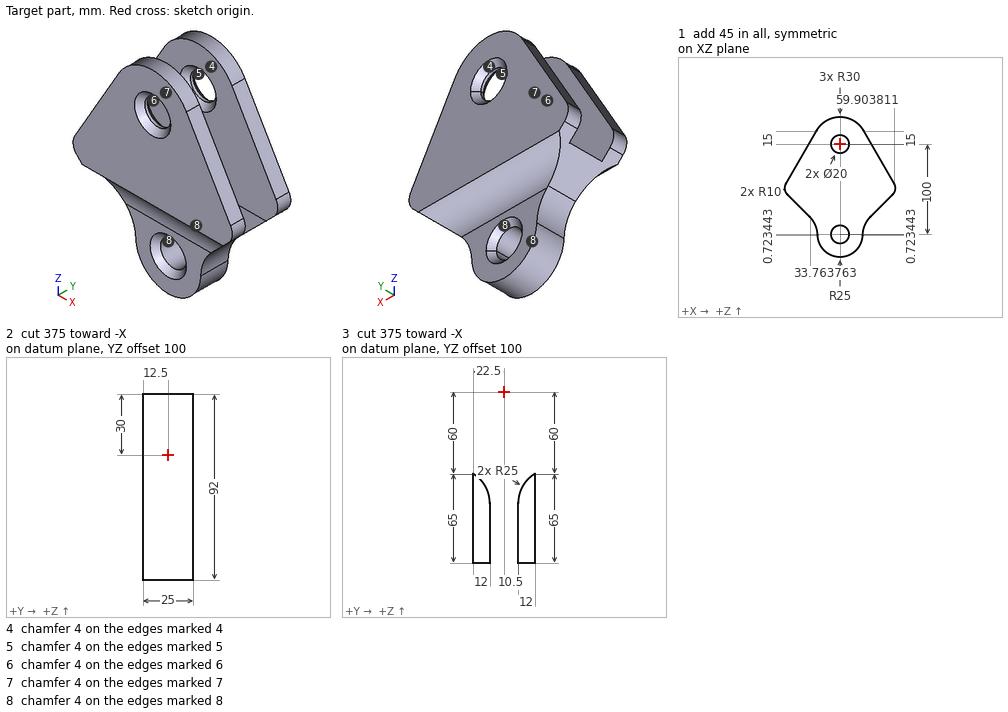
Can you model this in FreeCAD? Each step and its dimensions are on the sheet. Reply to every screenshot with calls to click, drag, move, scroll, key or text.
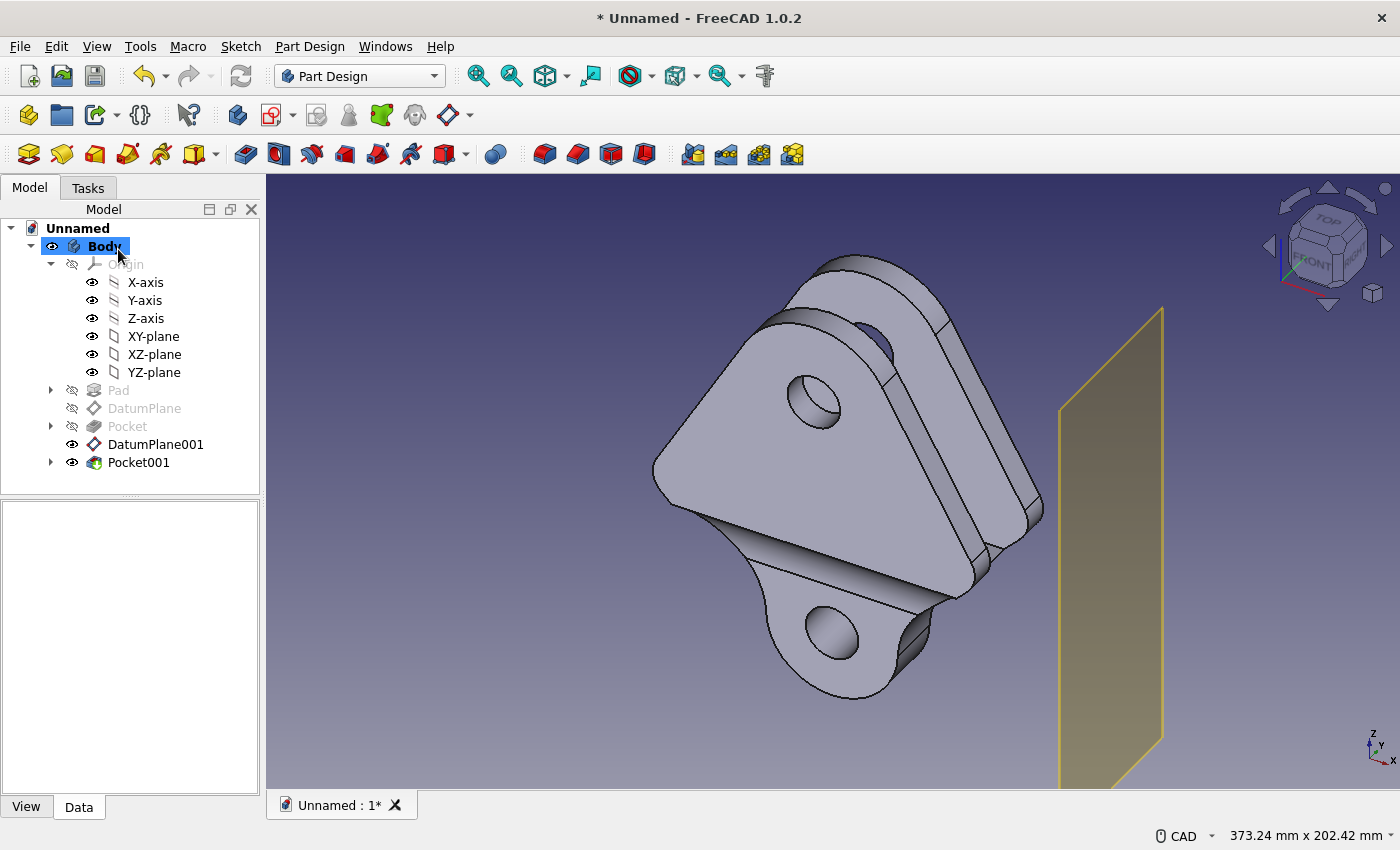
click(117, 444)
key(space)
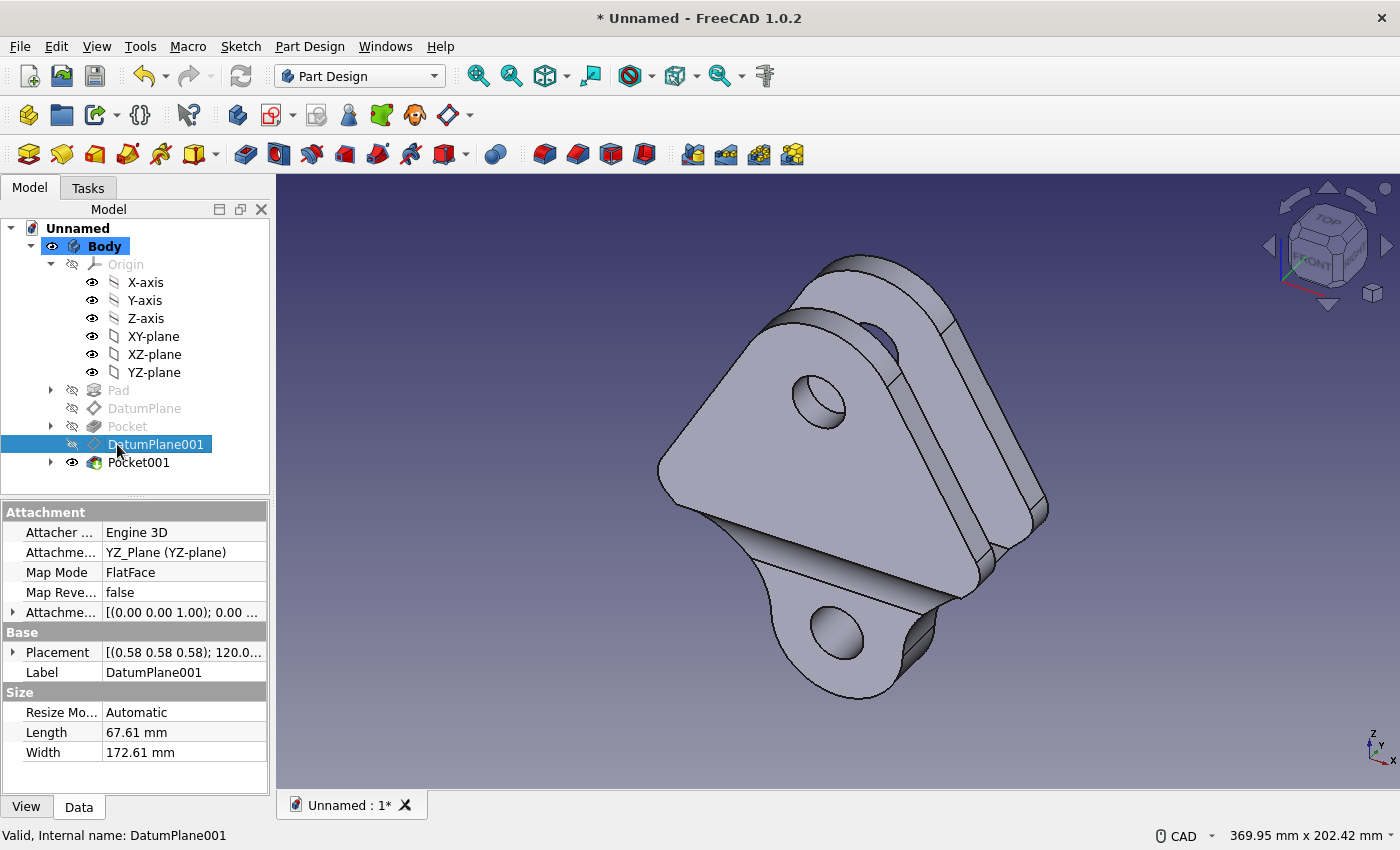
key(0)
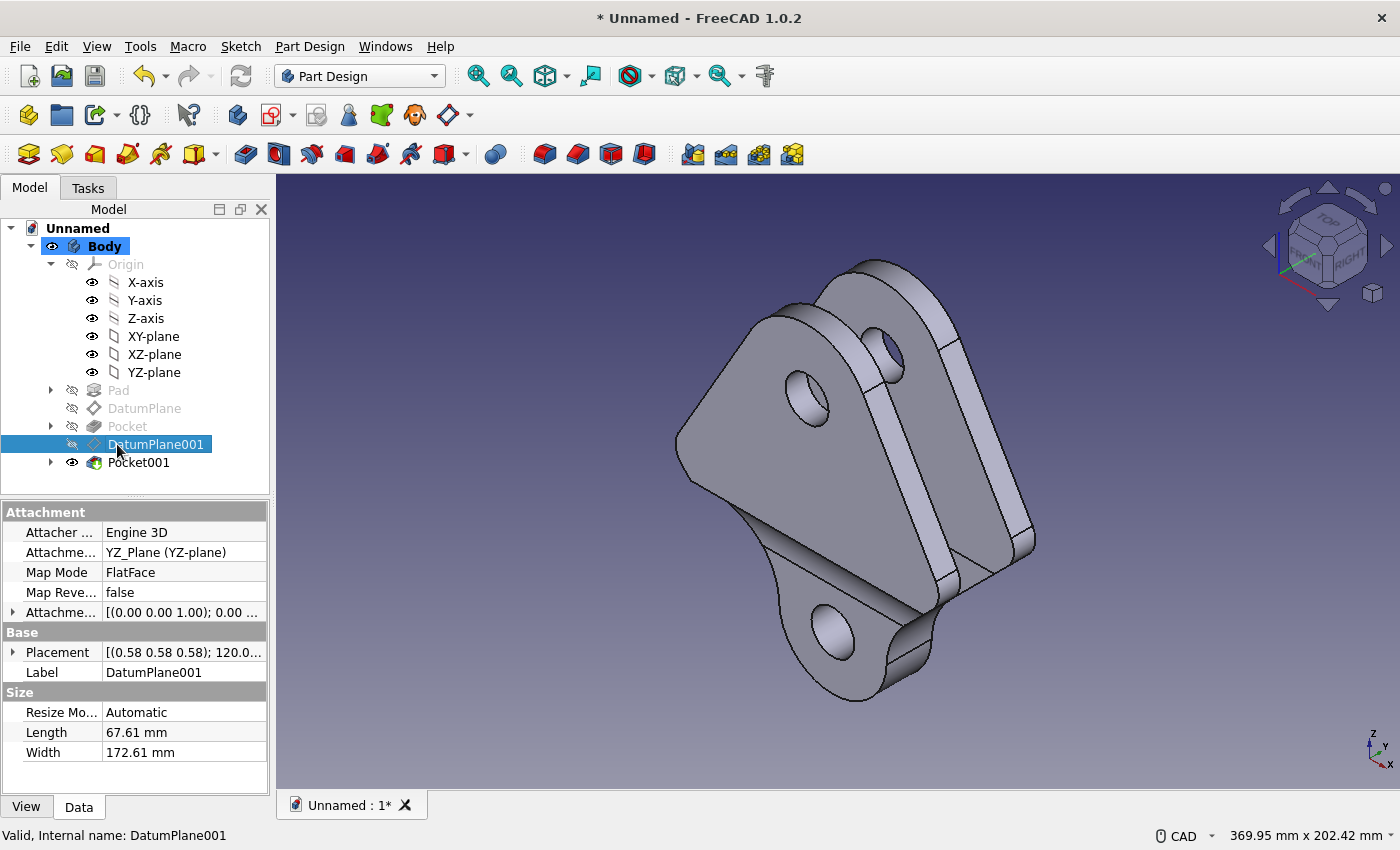
key(2)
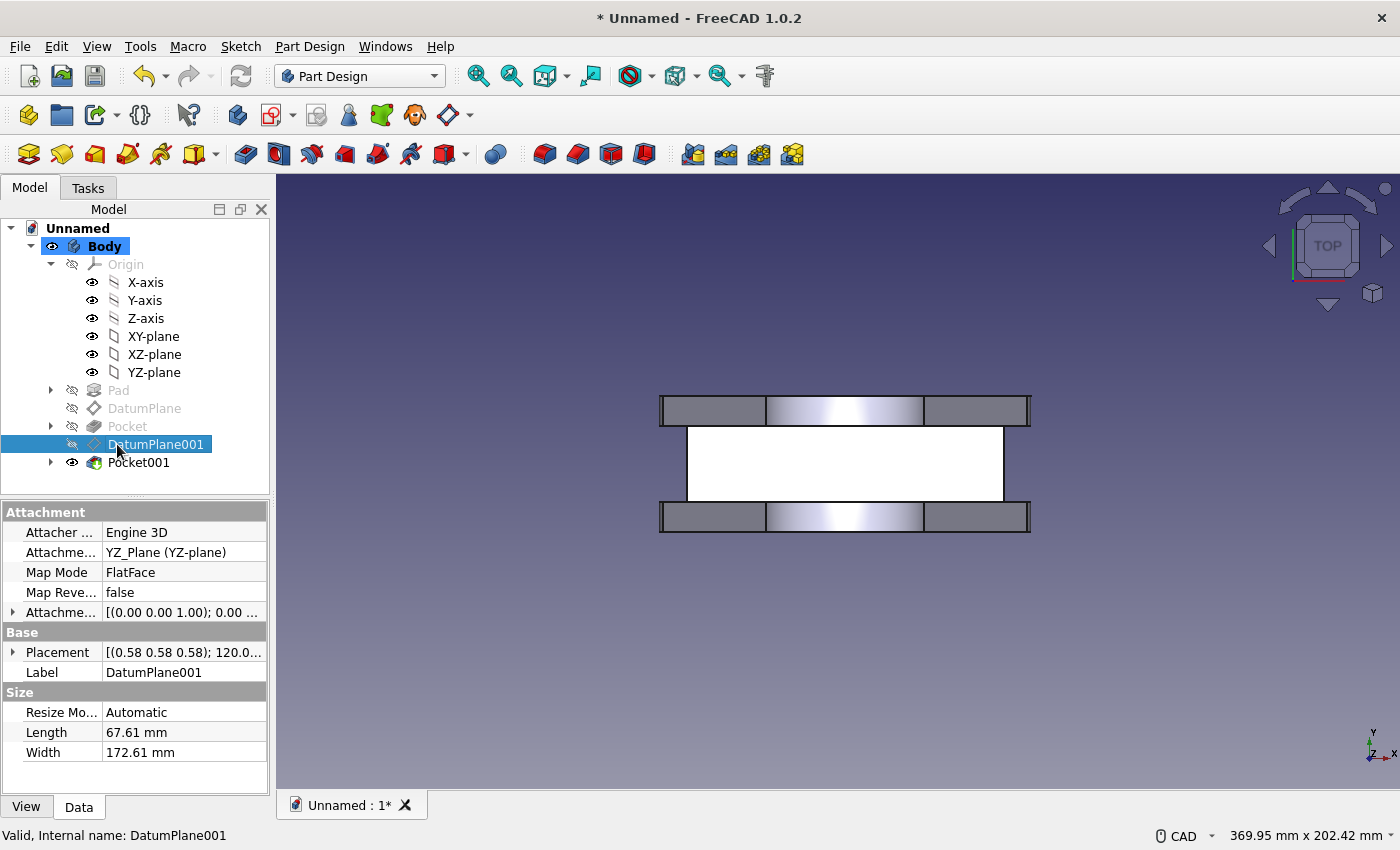
key(v)
key(f)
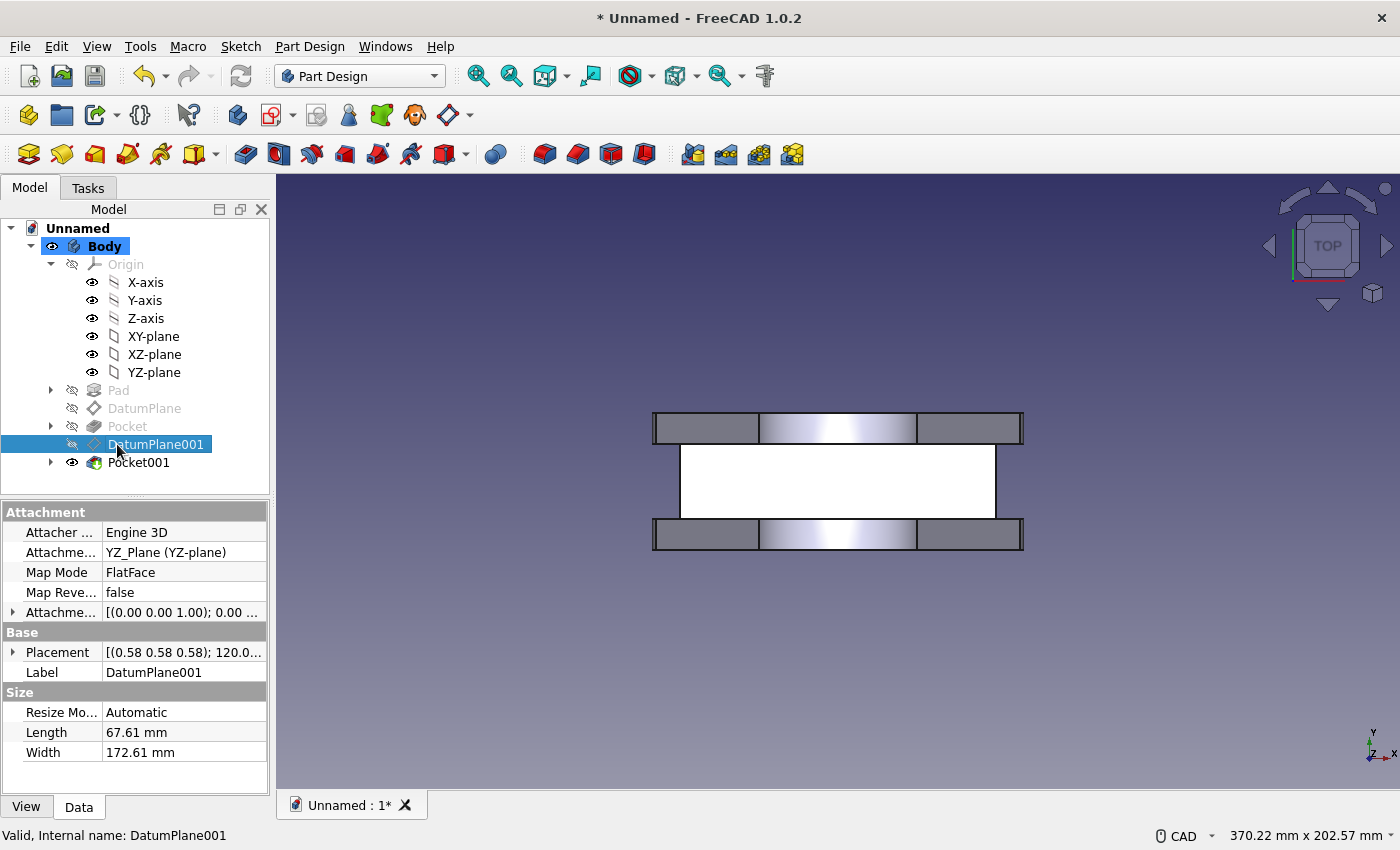
key(1)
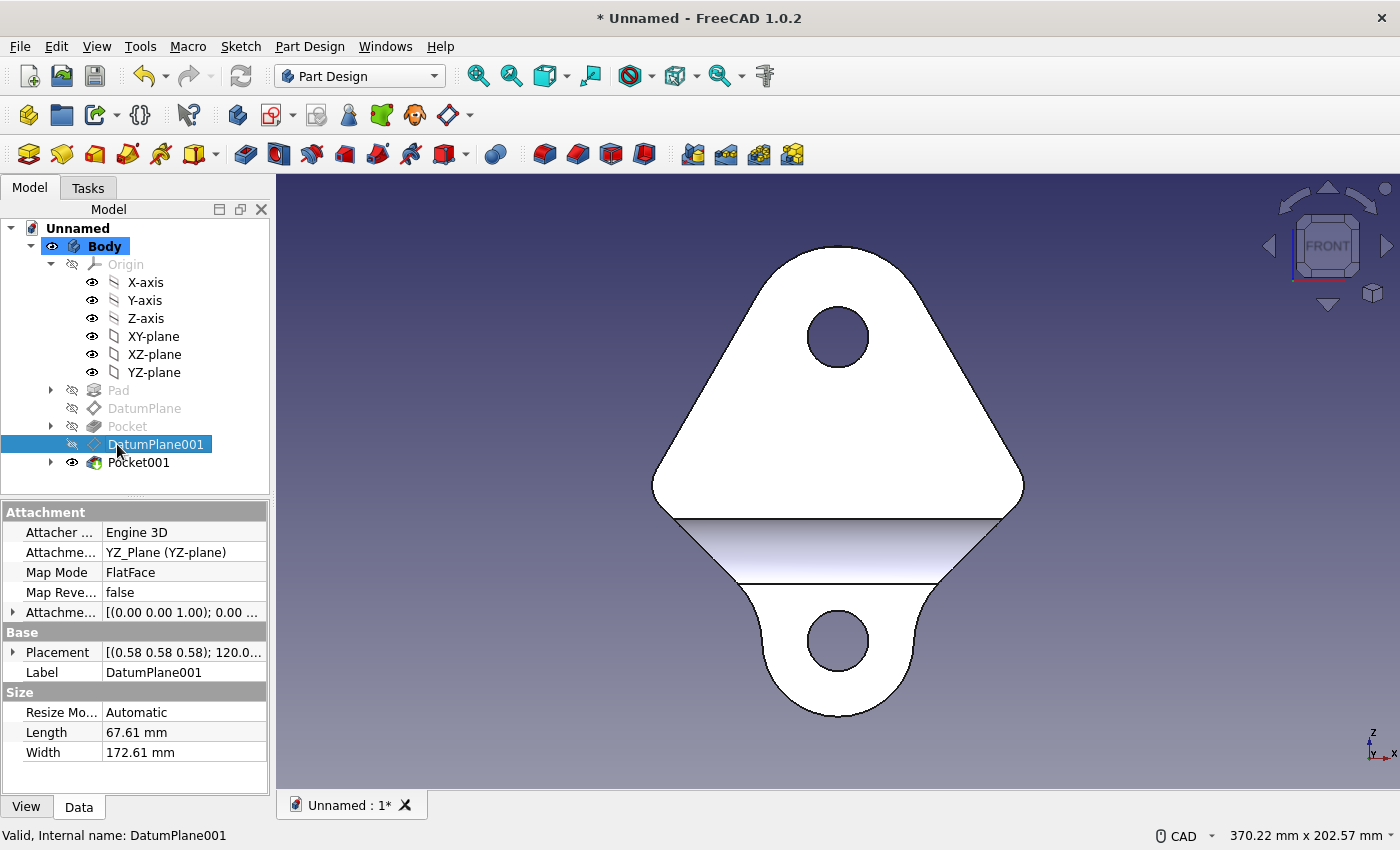
key(3)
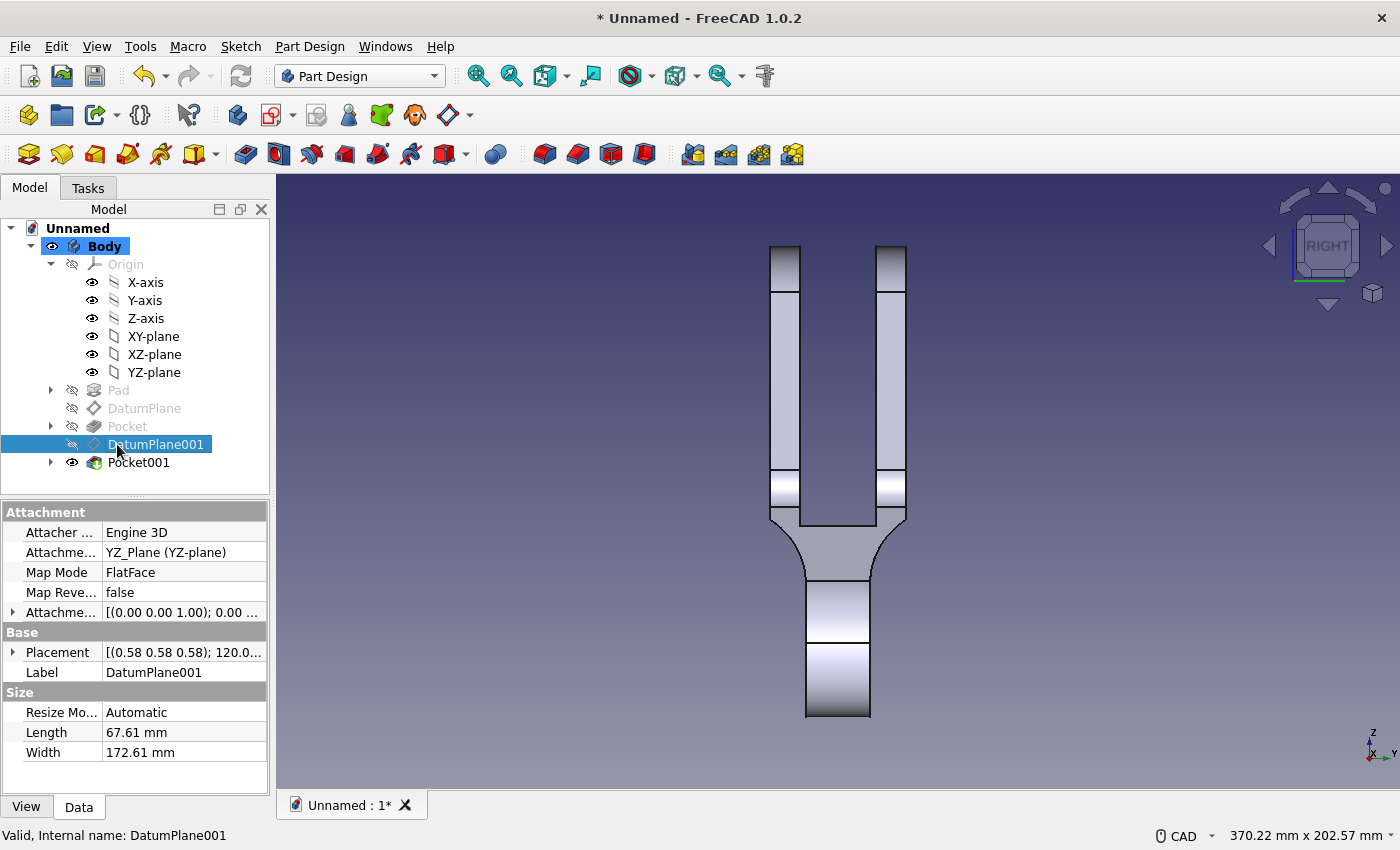
key(5)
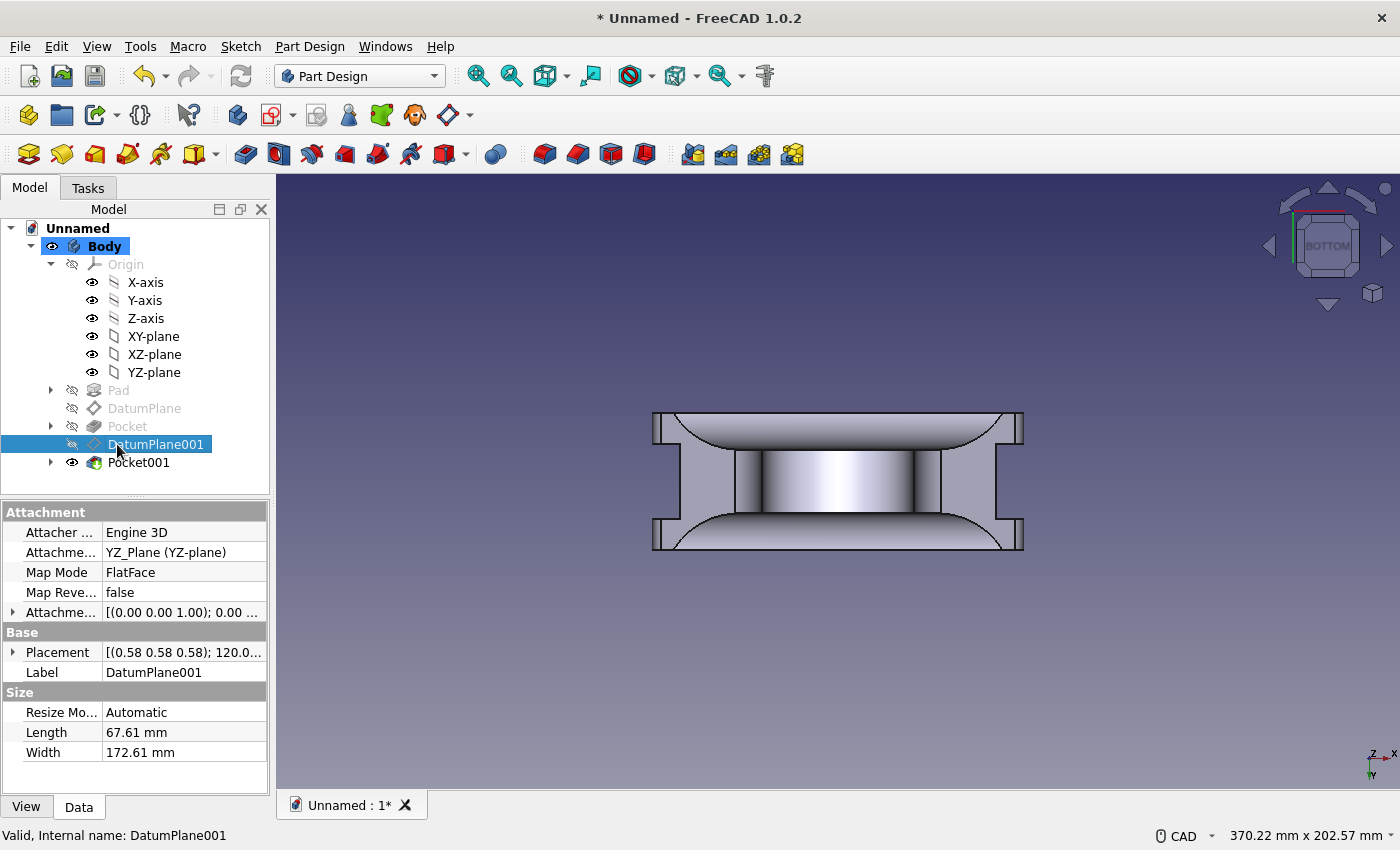
key(v)
key(f)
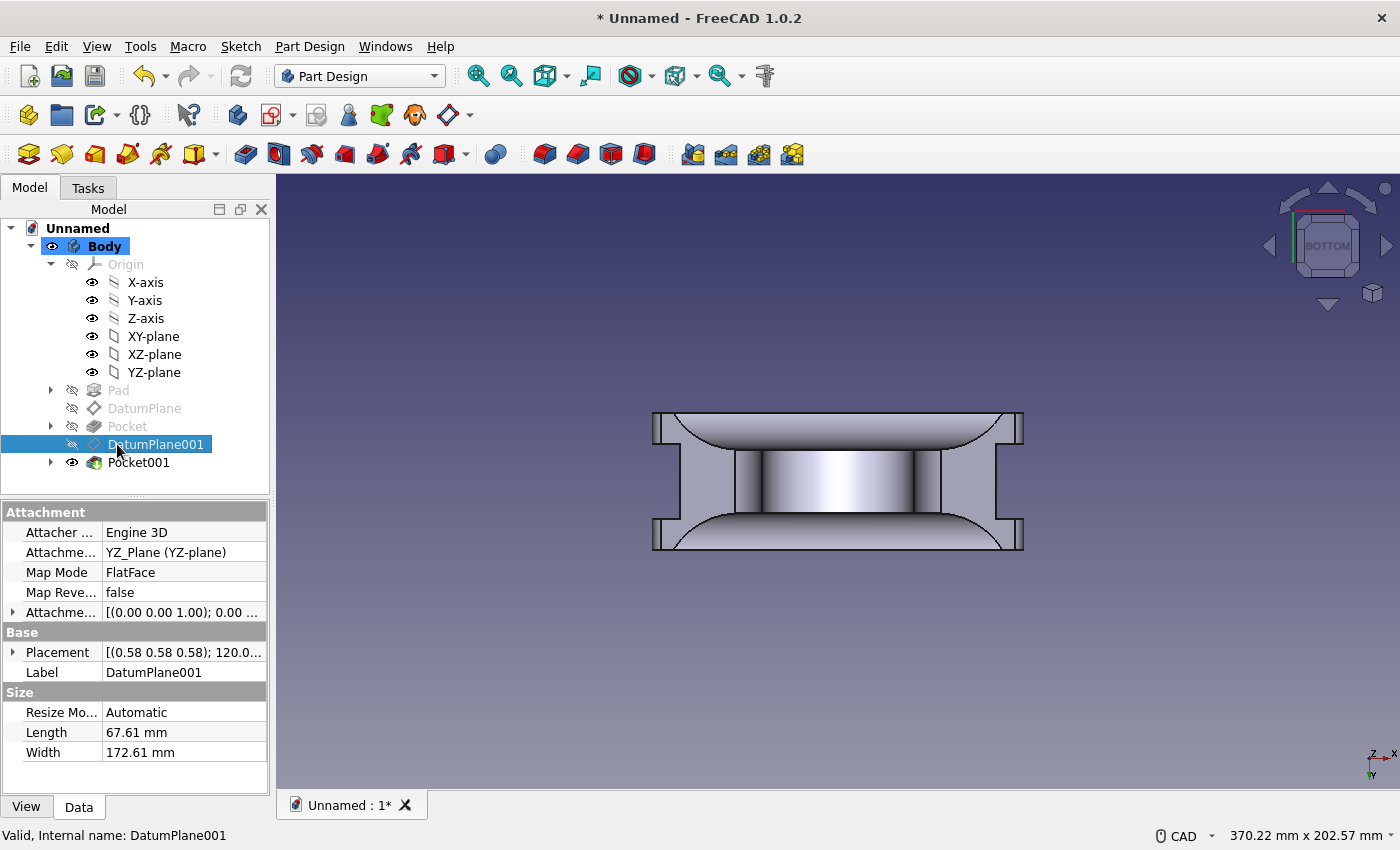
key(4)